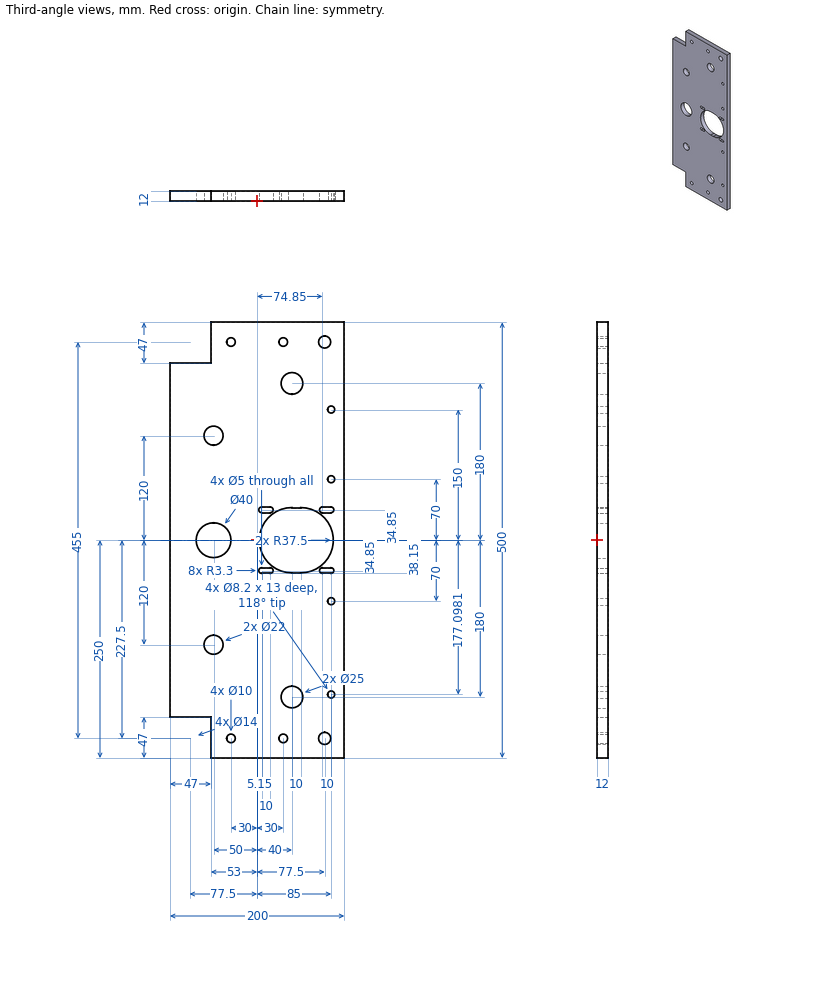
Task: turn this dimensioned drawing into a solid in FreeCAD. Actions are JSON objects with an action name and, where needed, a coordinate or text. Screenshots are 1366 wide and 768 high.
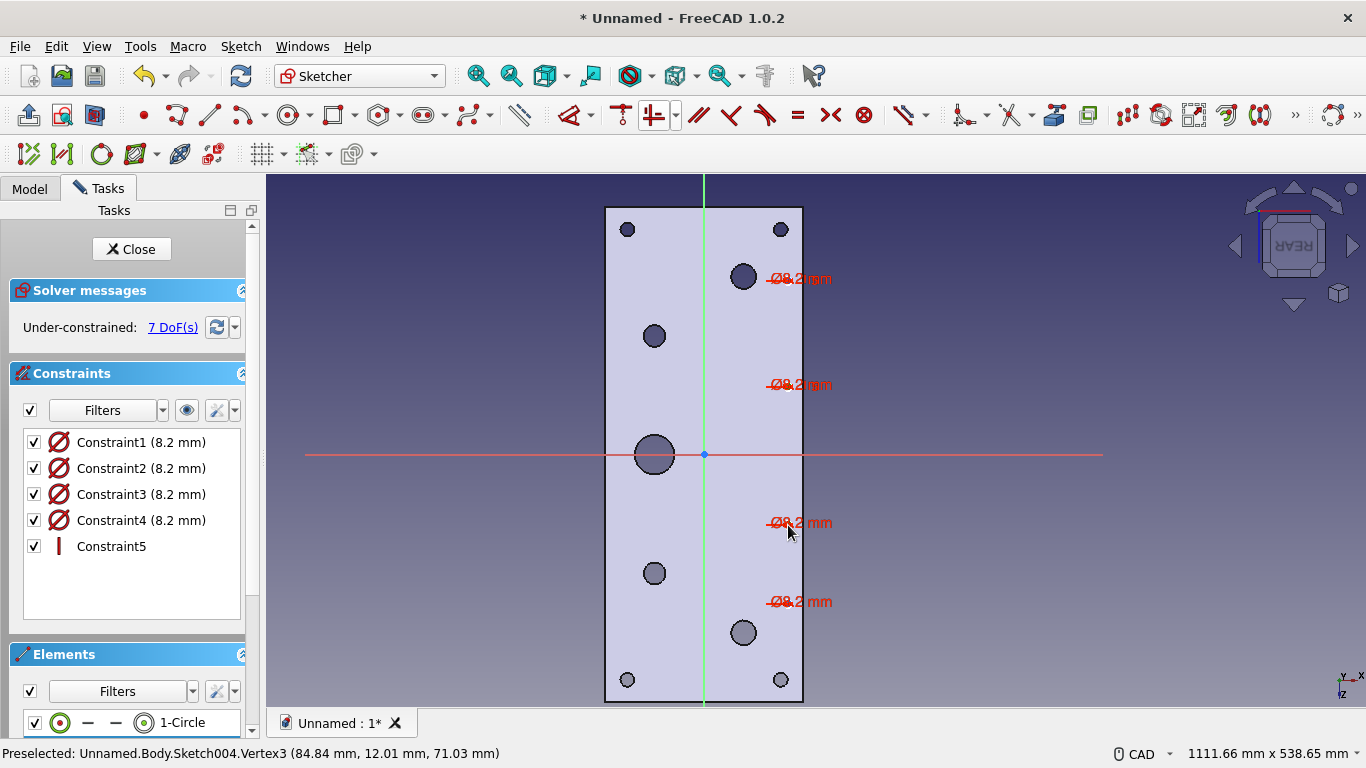
{"action": "key", "text": "v"}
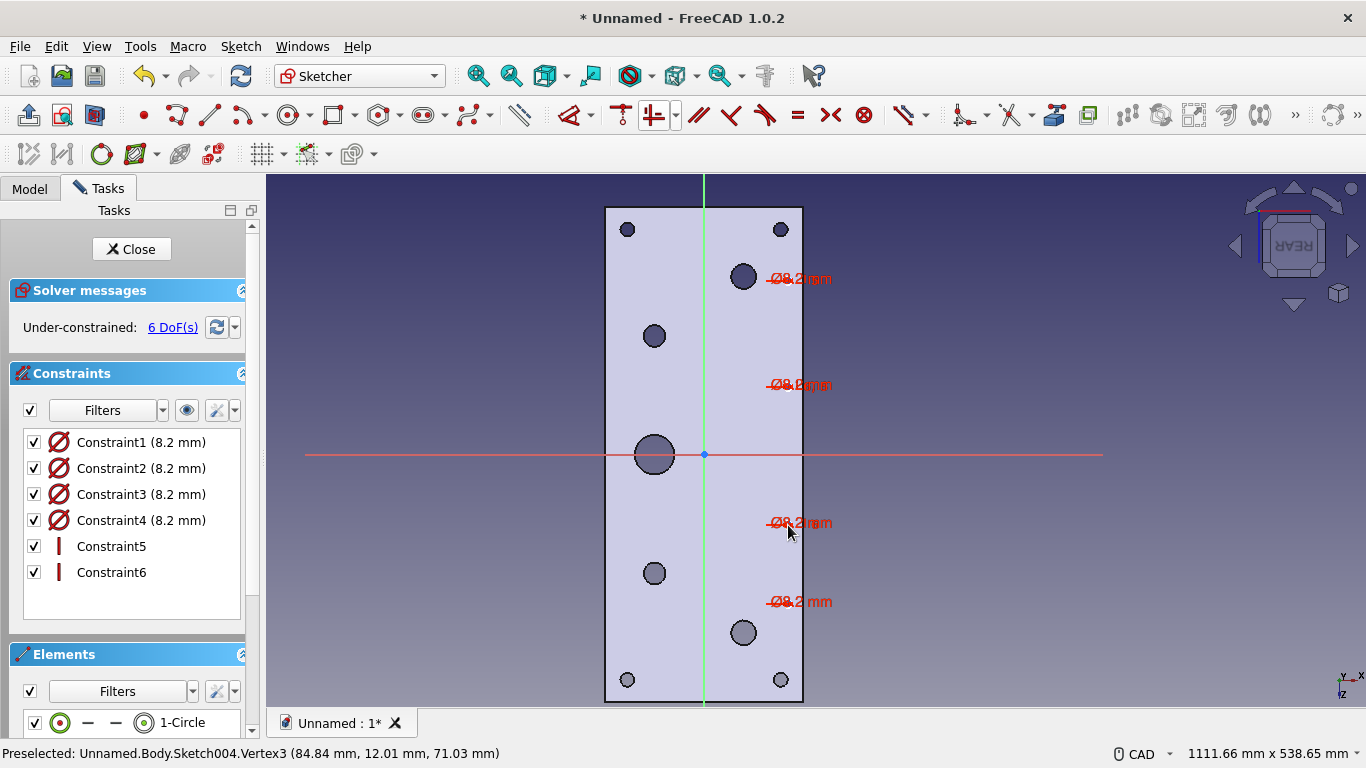
{"action": "left_click", "coordinate": [788, 525]}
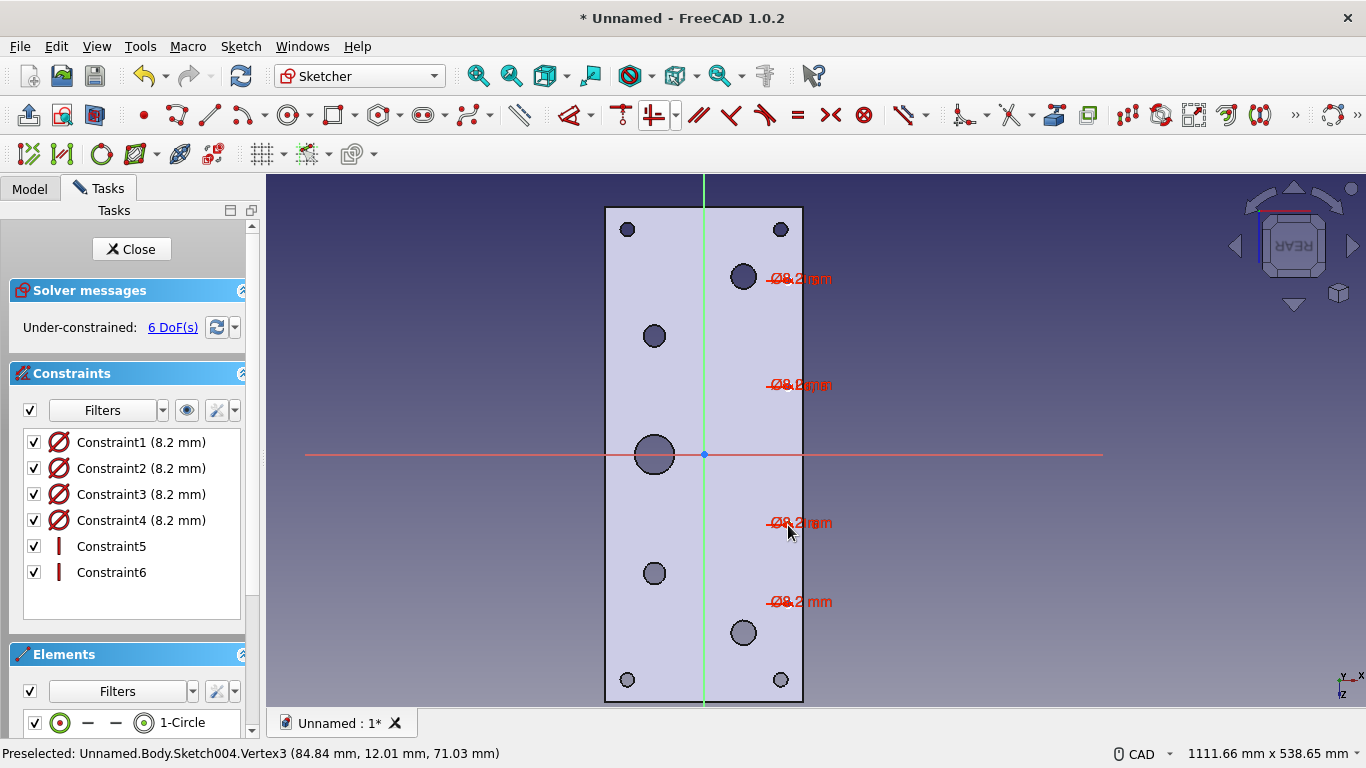
{"action": "left_click", "coordinate": [788, 604]}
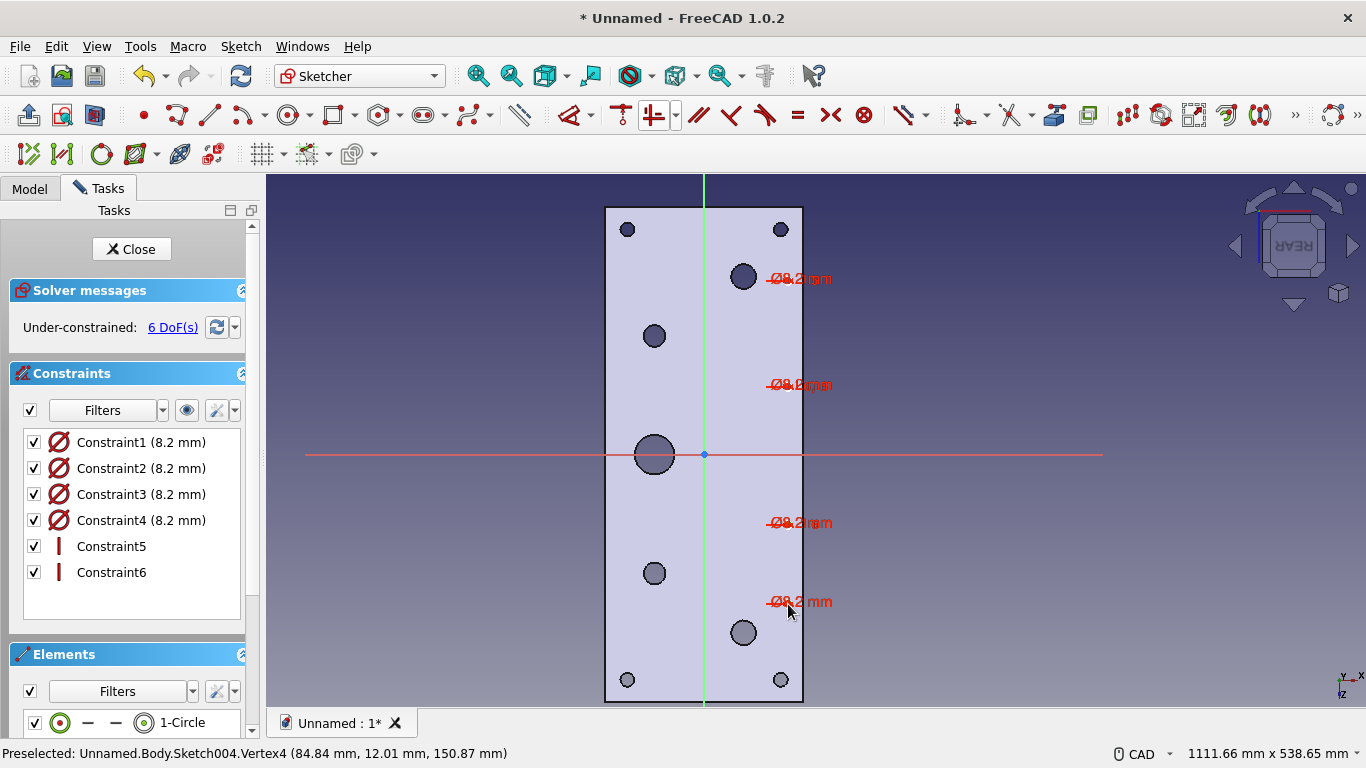
{"action": "key", "text": "v"}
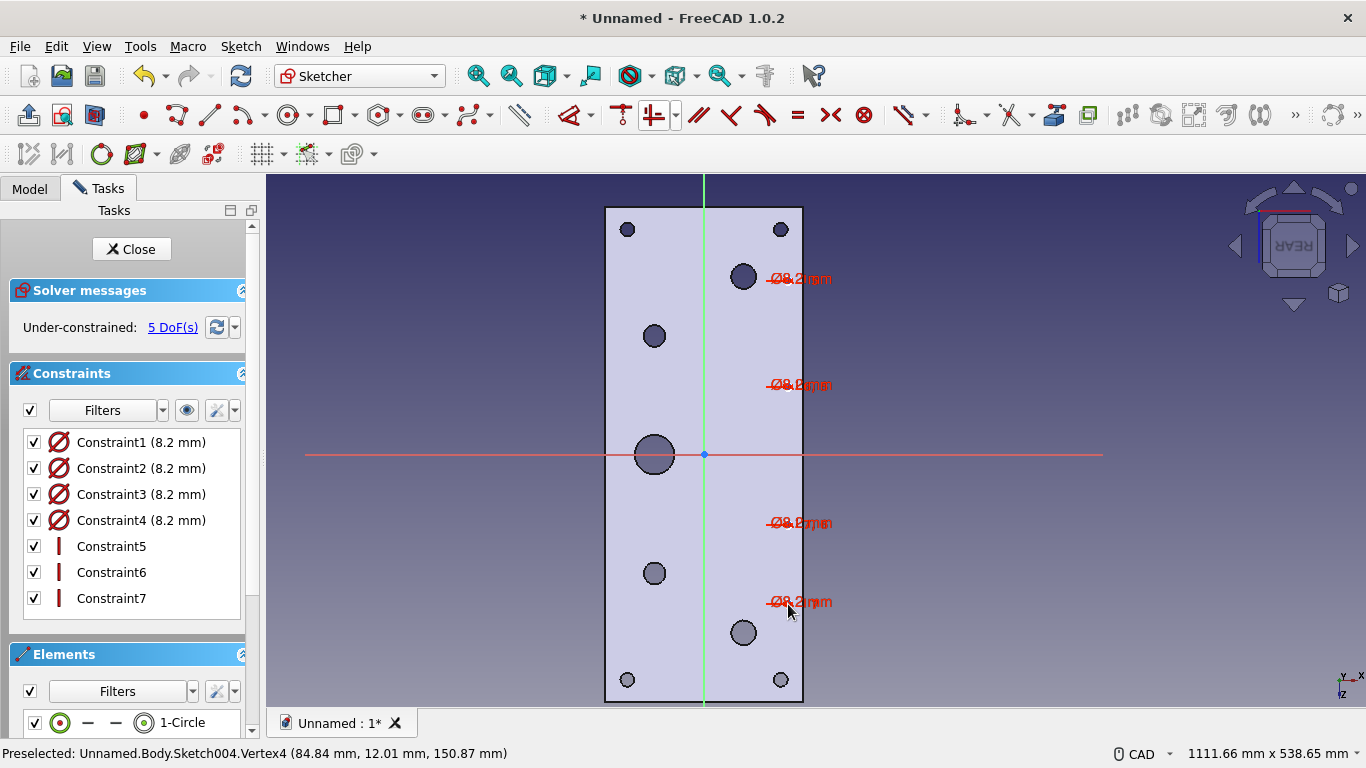
{"action": "key", "text": "d"}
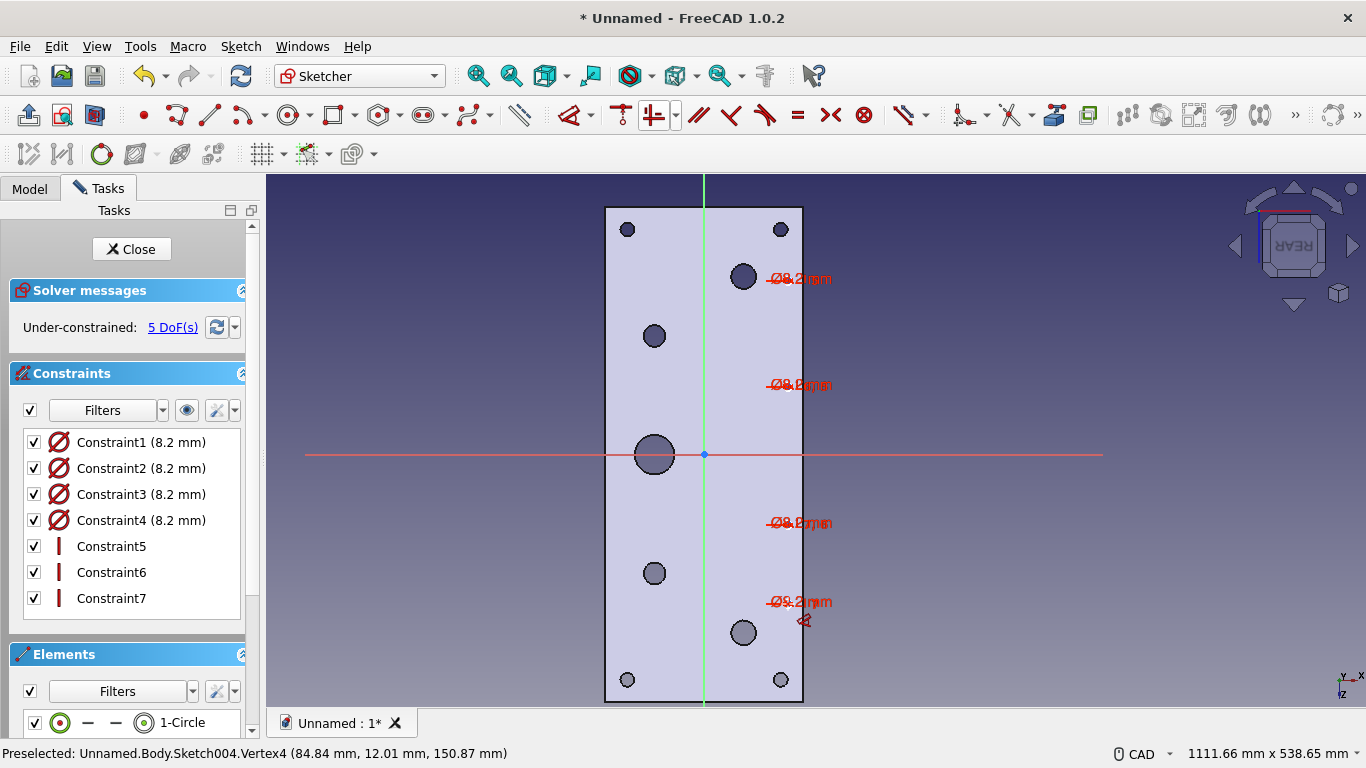
{"action": "left_click", "coordinate": [788, 281]}
{"action": "left_click", "coordinate": [746, 247]}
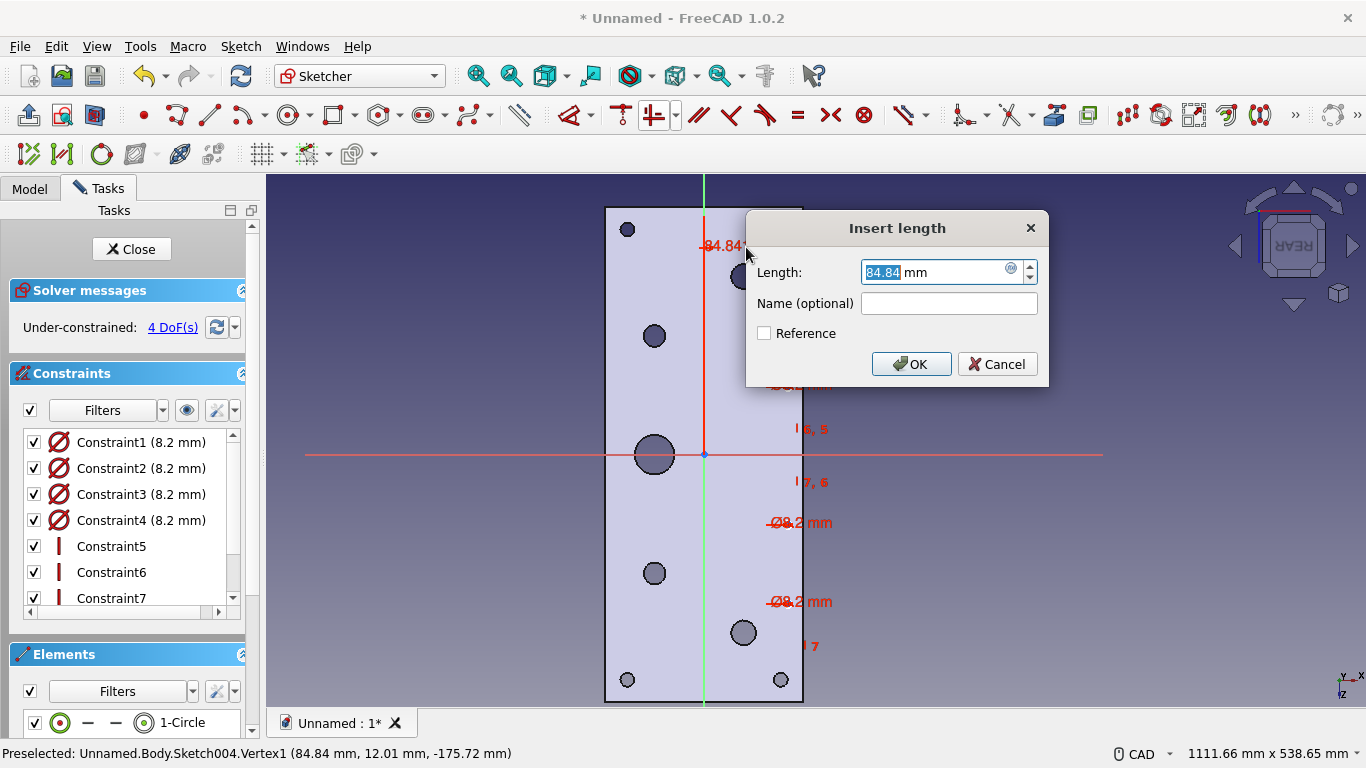
{"action": "type", "text": "85"}
{"action": "key", "text": "Return"}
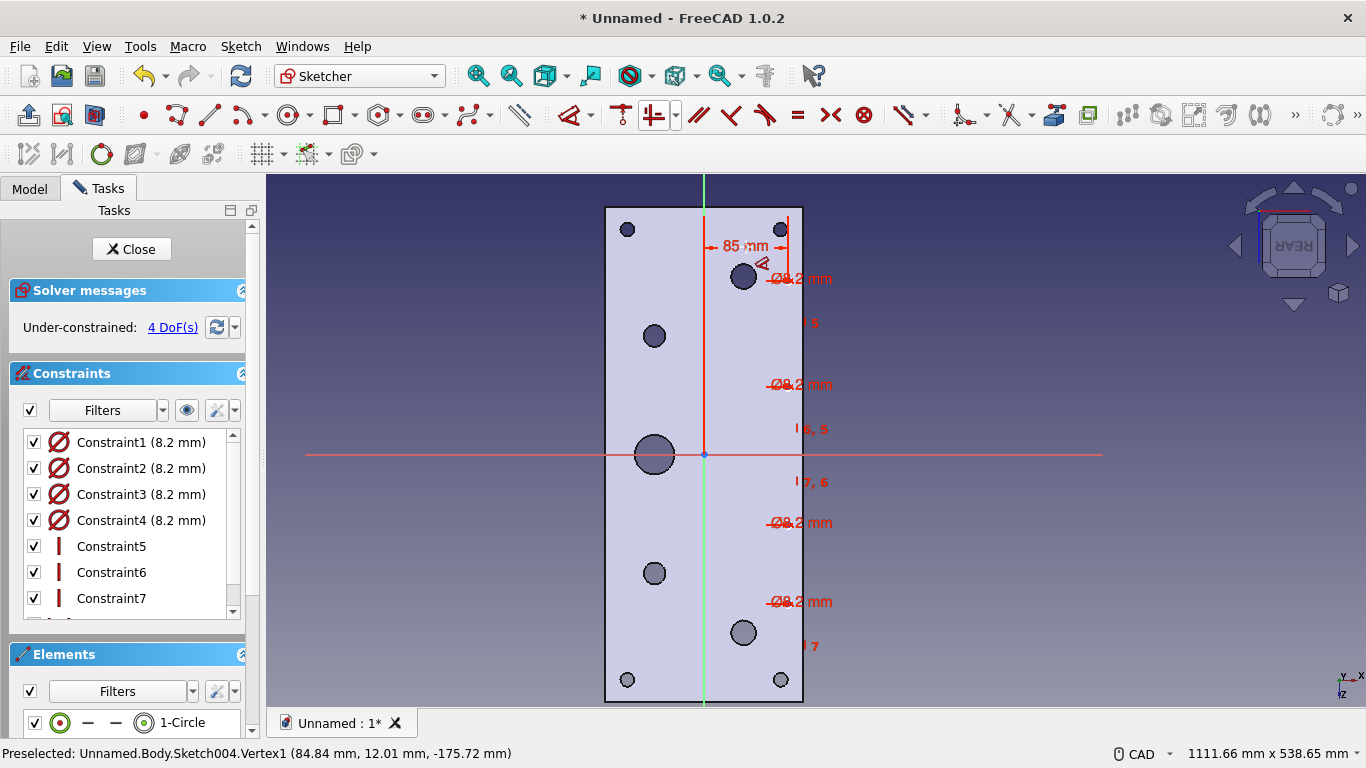
{"action": "left_click", "coordinate": [788, 387]}
{"action": "left_click", "coordinate": [670, 421]}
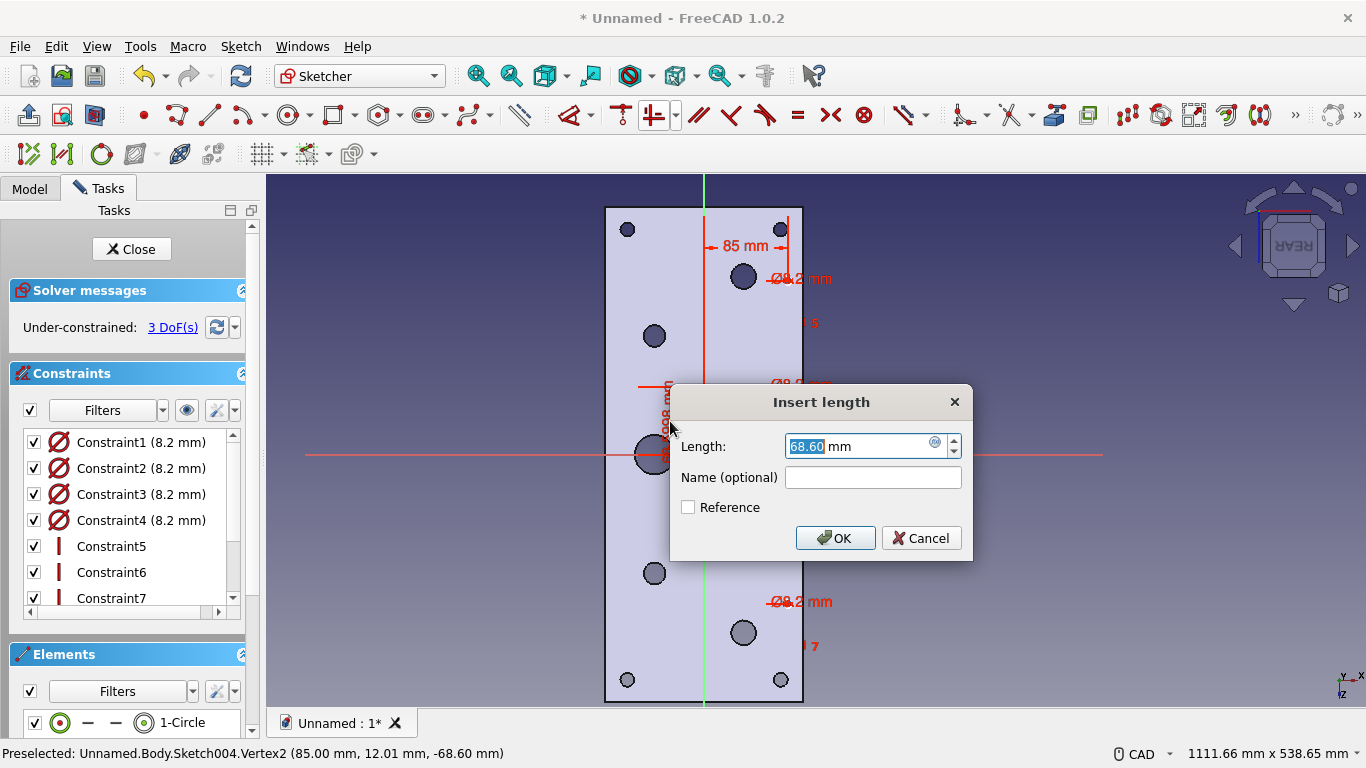
{"action": "type", "text": "70"}
{"action": "key", "text": "Return"}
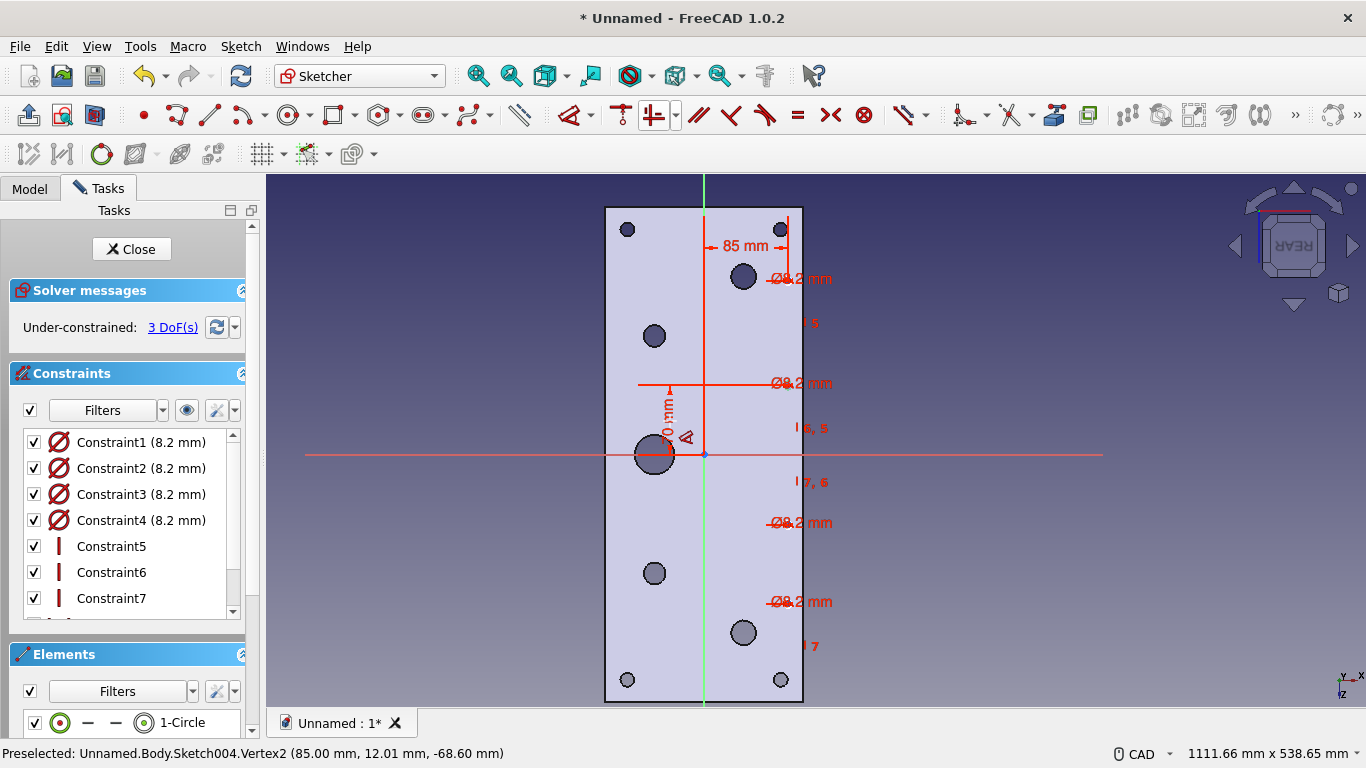
{"action": "left_click", "coordinate": [788, 525]}
{"action": "left_click", "coordinate": [670, 490]}